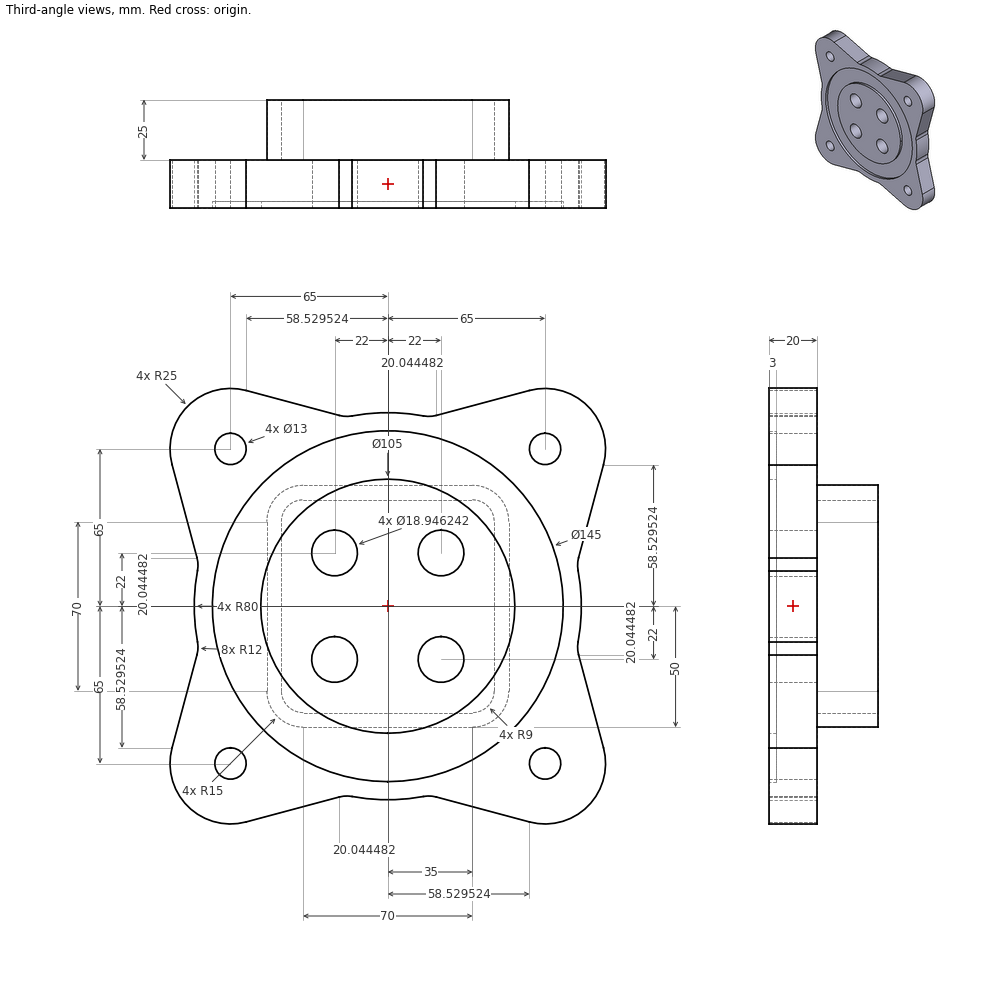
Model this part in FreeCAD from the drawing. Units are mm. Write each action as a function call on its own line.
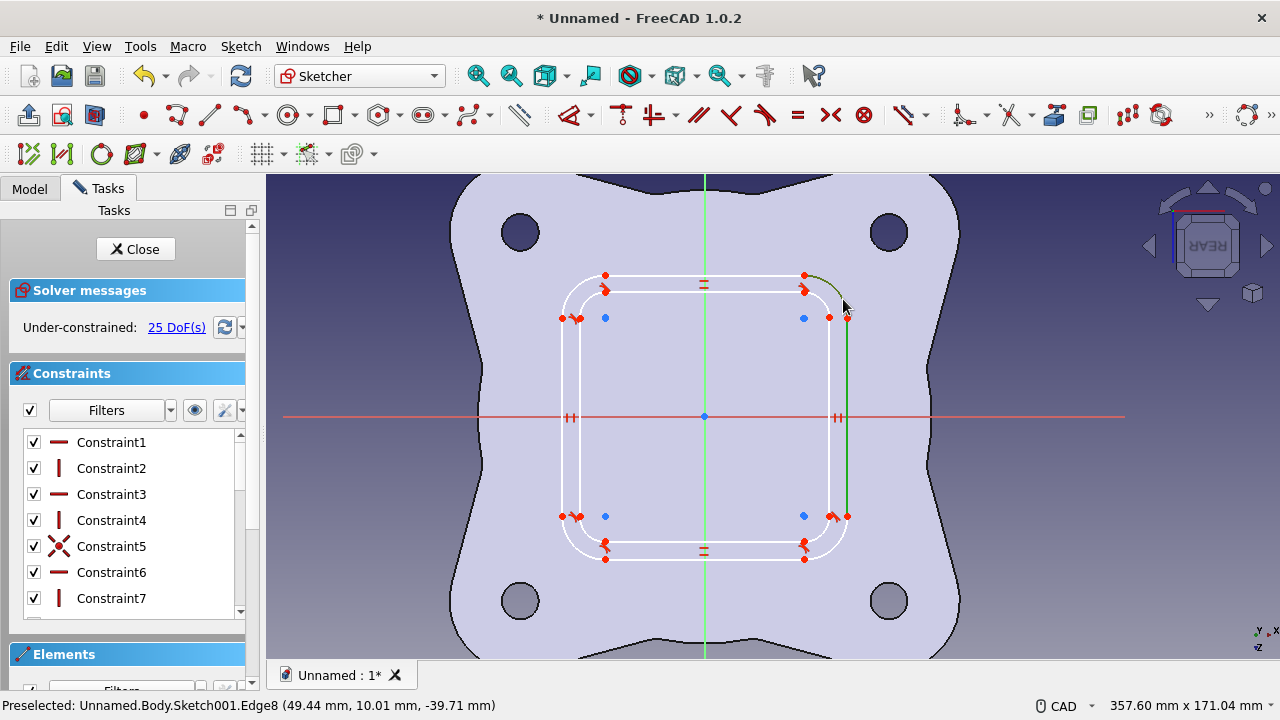
click(765, 116)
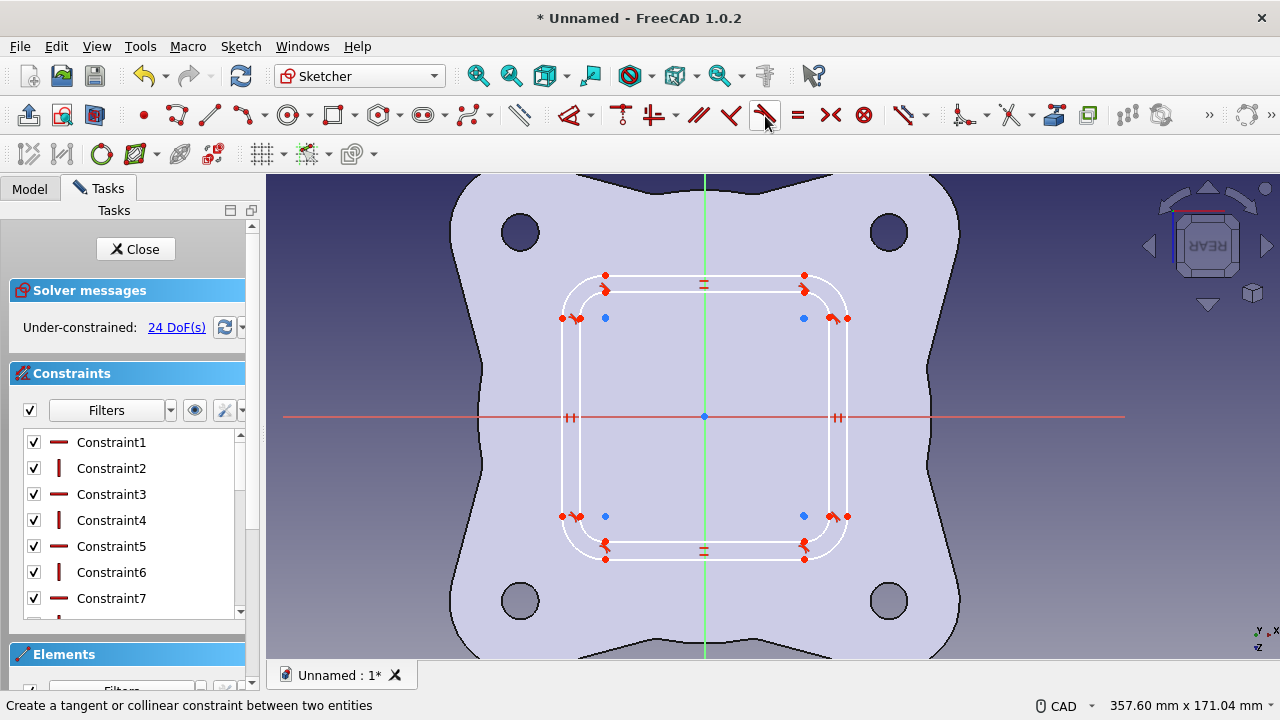
click(665, 292)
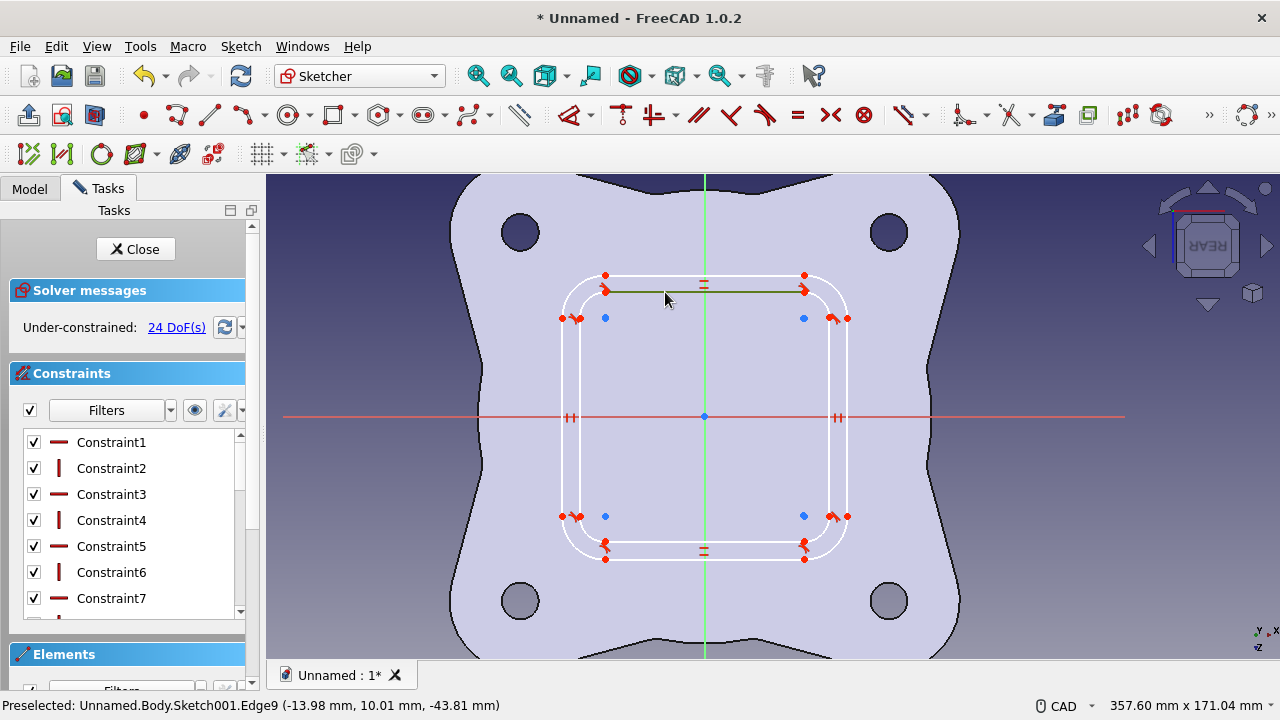
click(827, 306)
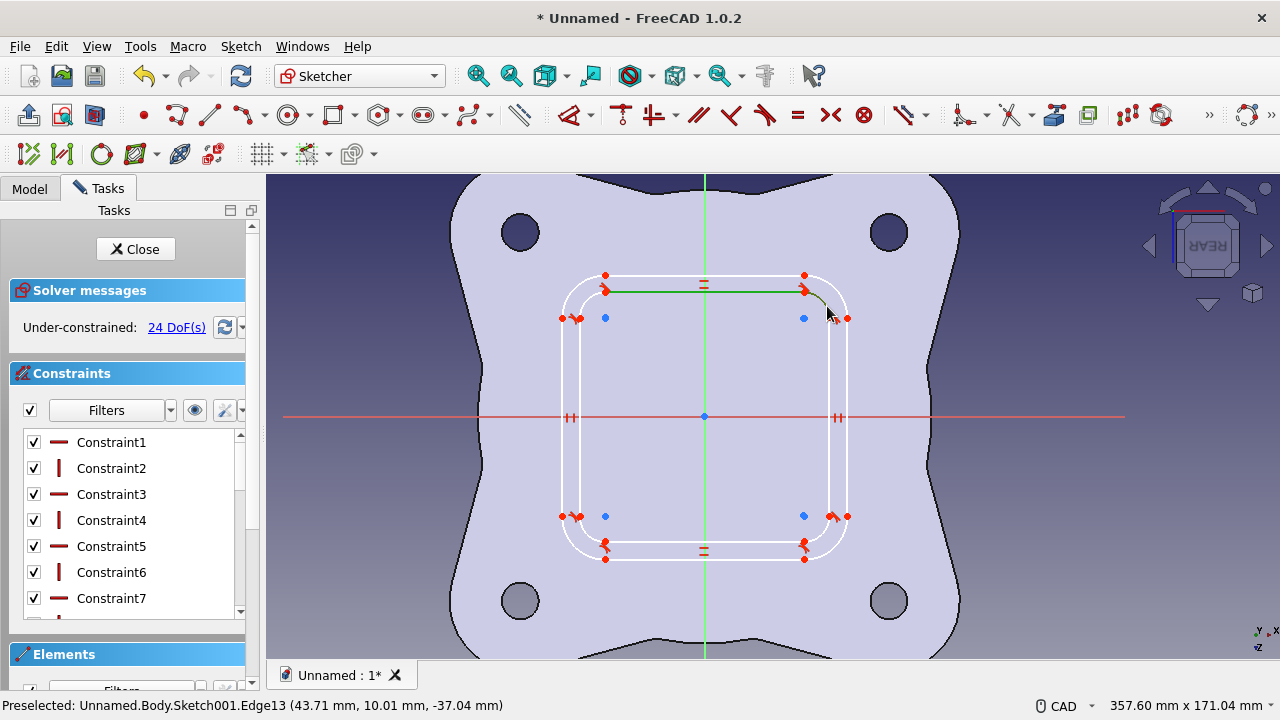
click(765, 116)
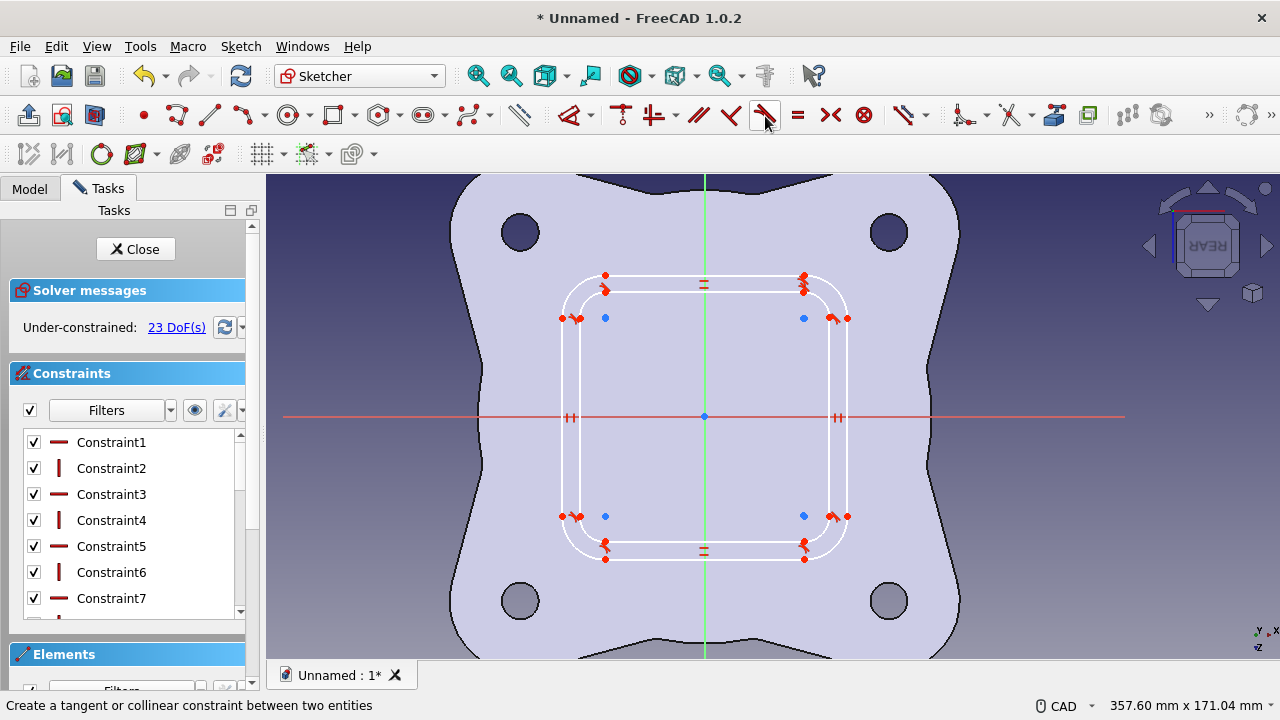
click(665, 292)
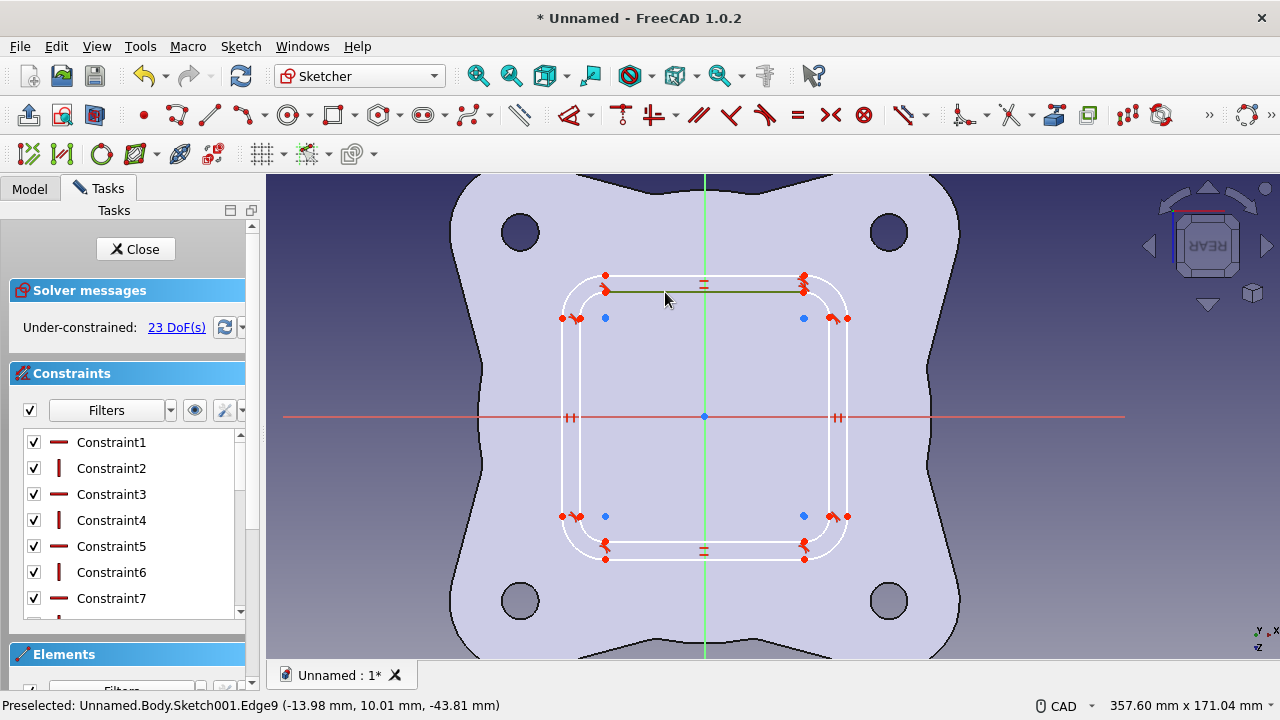
click(594, 295)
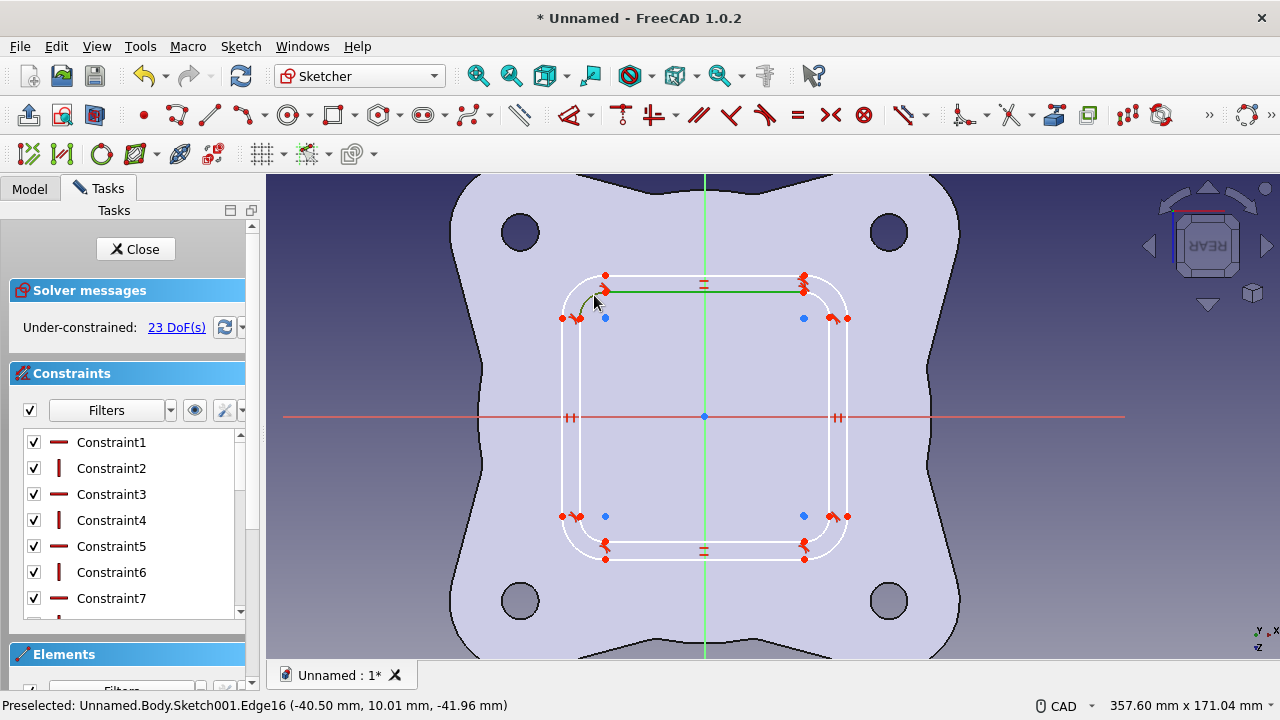
click(765, 116)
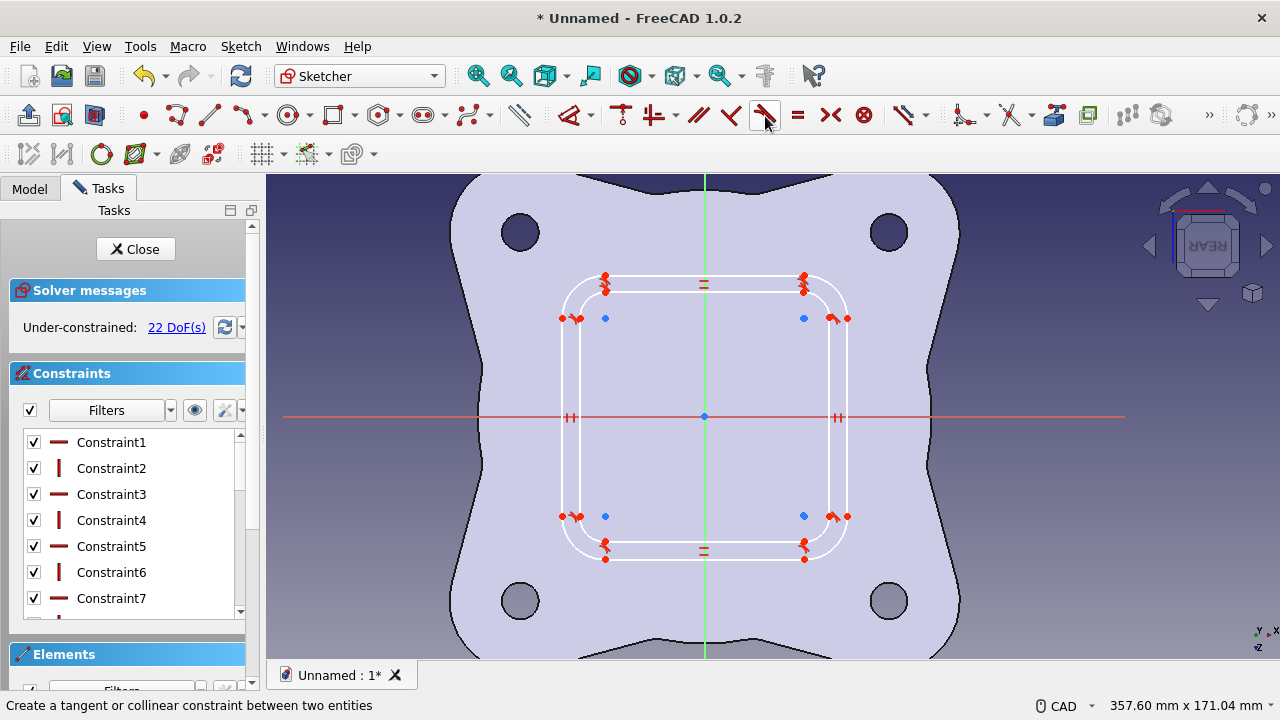
click(829, 377)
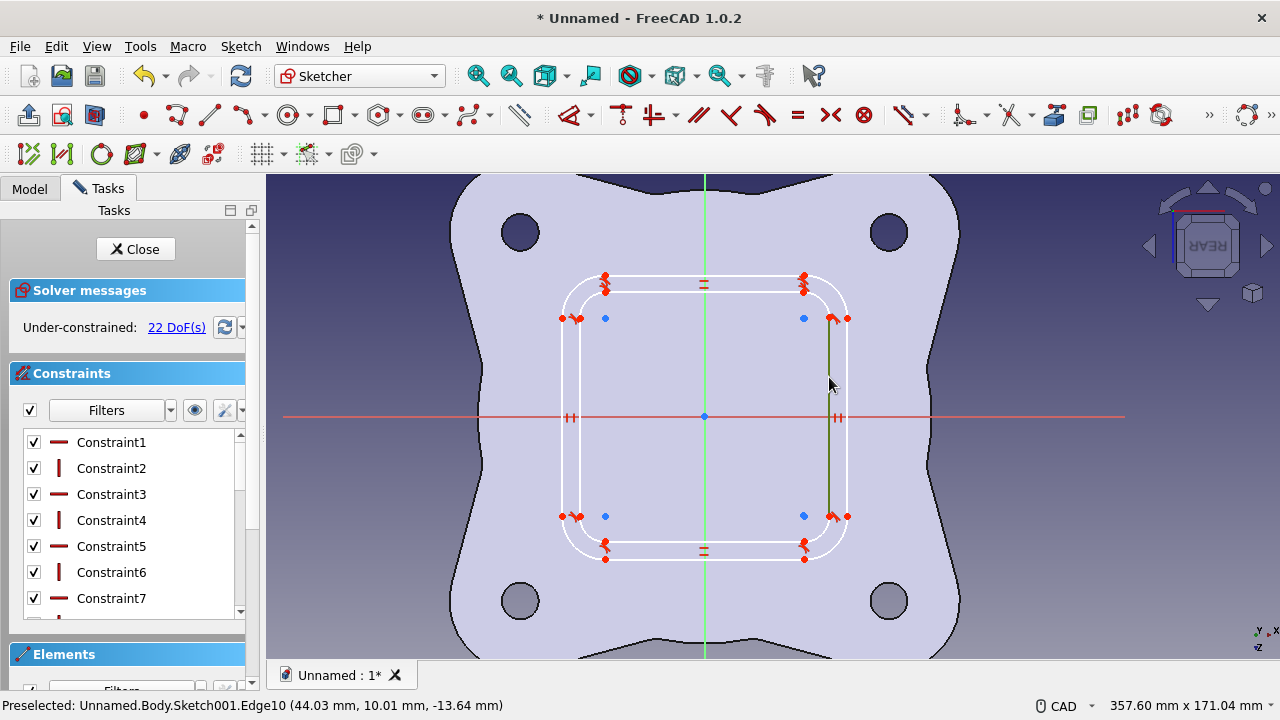
click(826, 306)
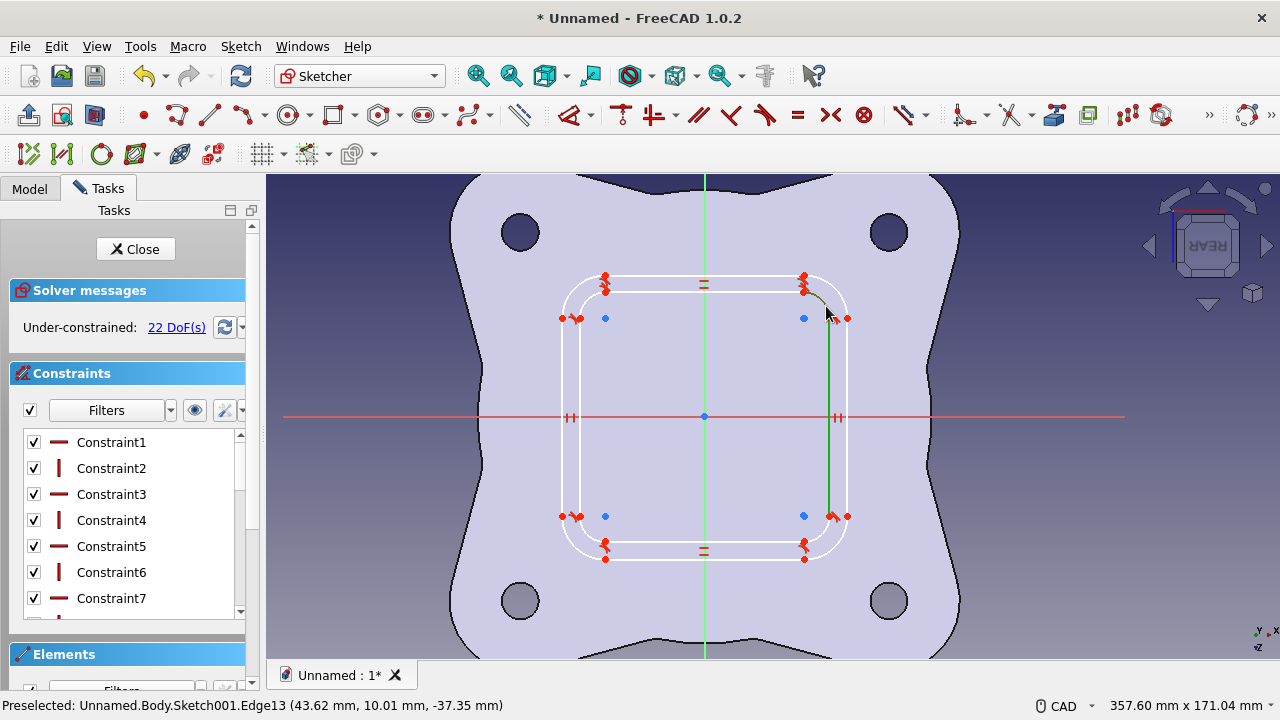
click(765, 116)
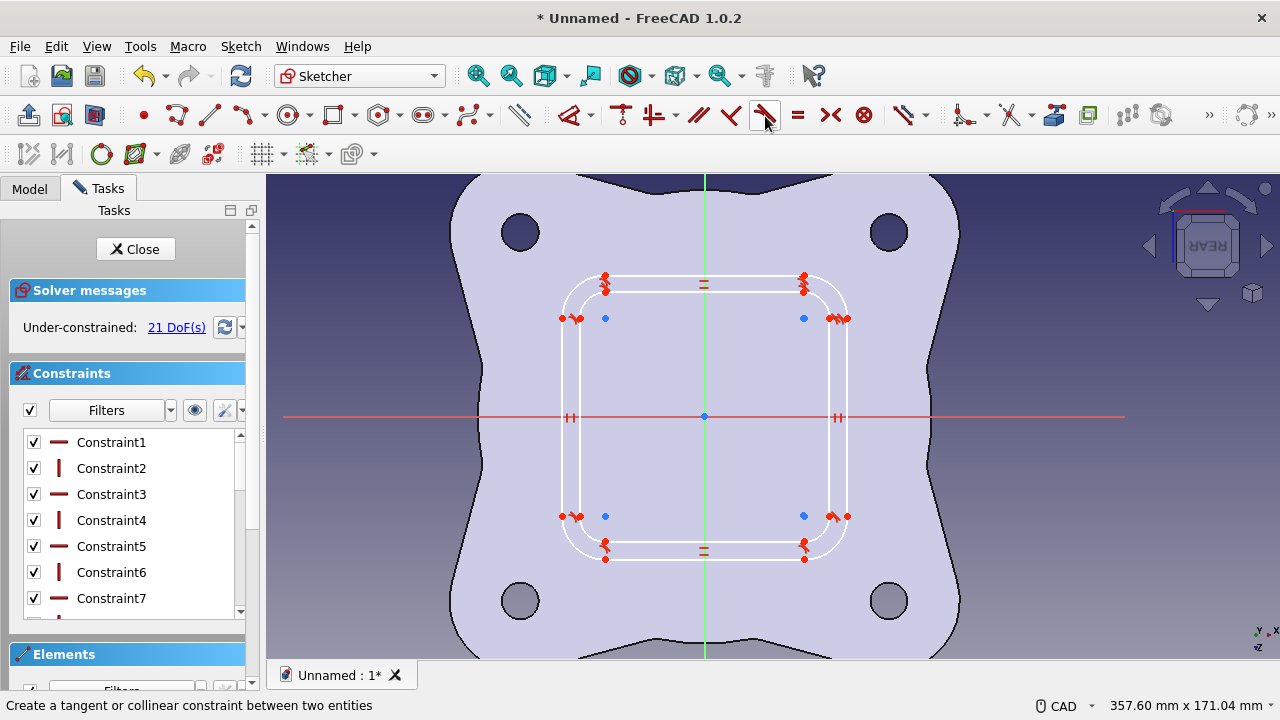
click(829, 378)